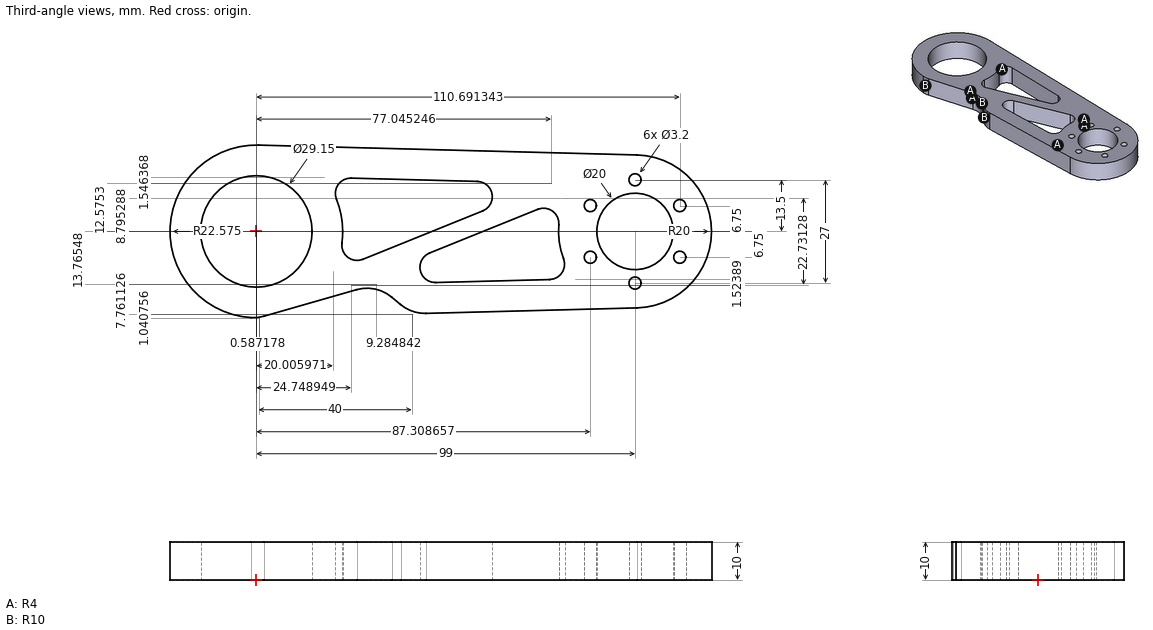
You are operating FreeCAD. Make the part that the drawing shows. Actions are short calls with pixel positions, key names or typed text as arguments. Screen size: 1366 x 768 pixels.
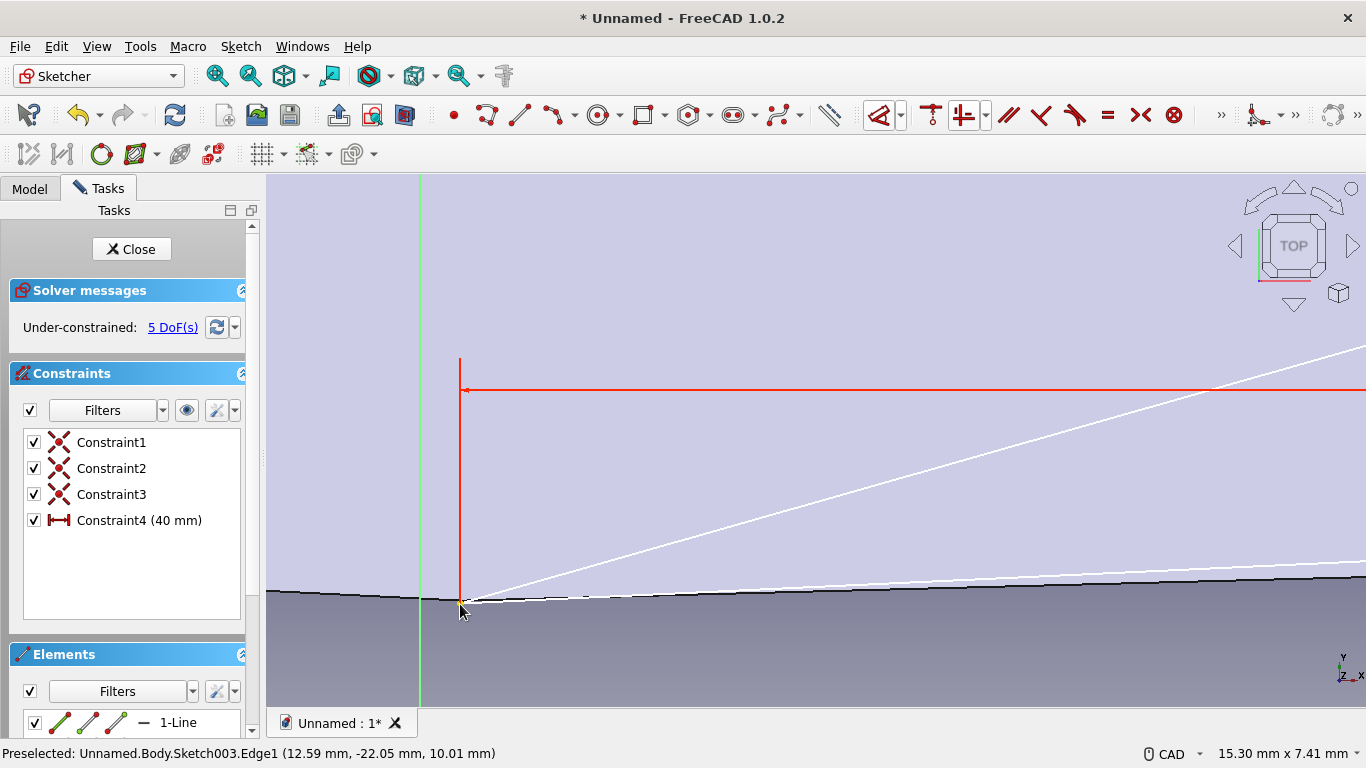
click(460, 604)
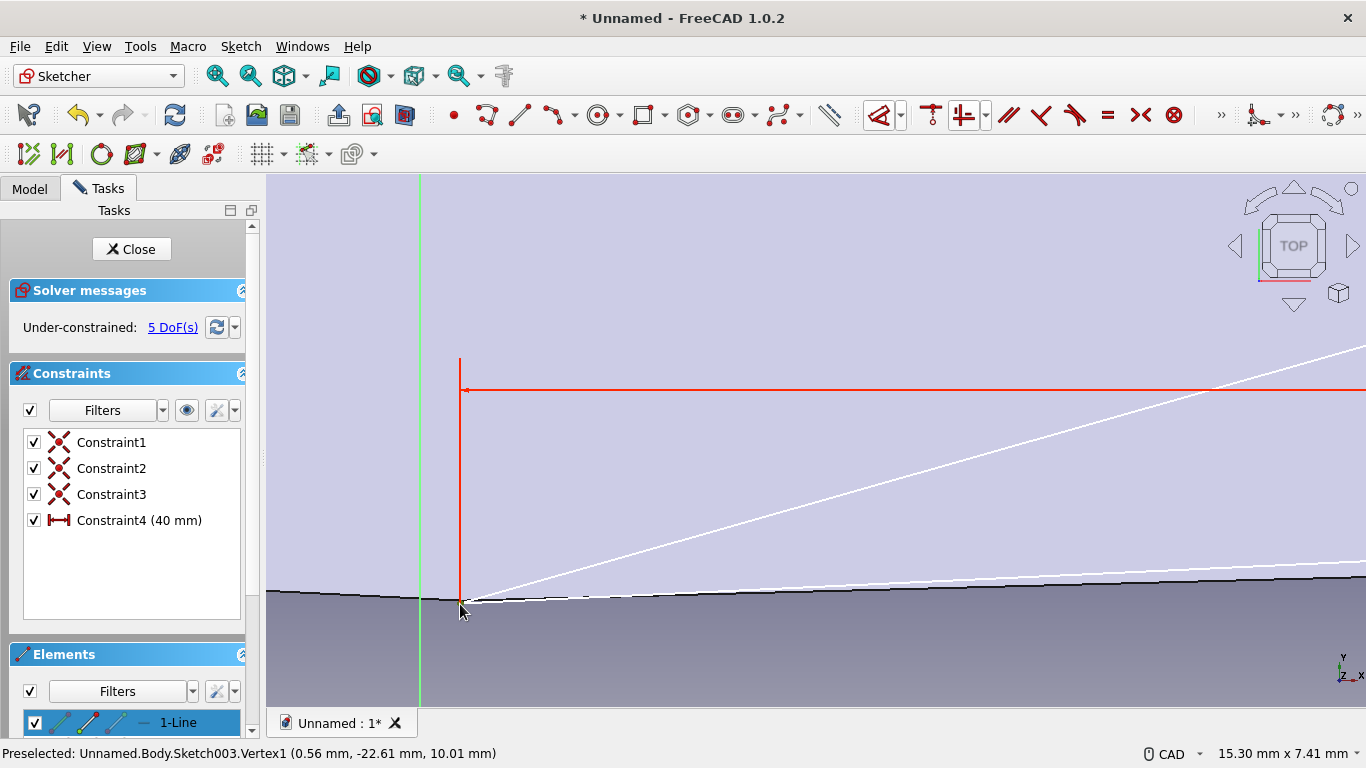
key(l)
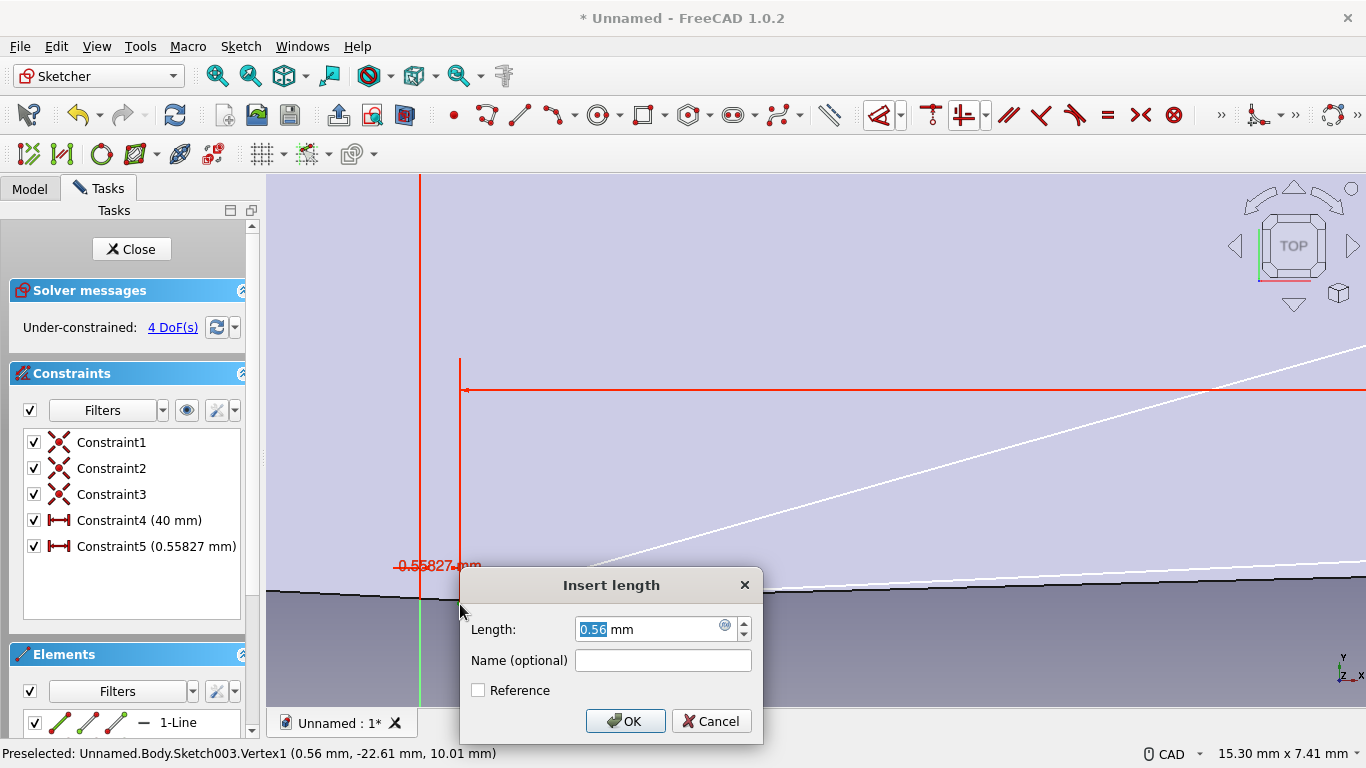
text(0.587178)
key(Return)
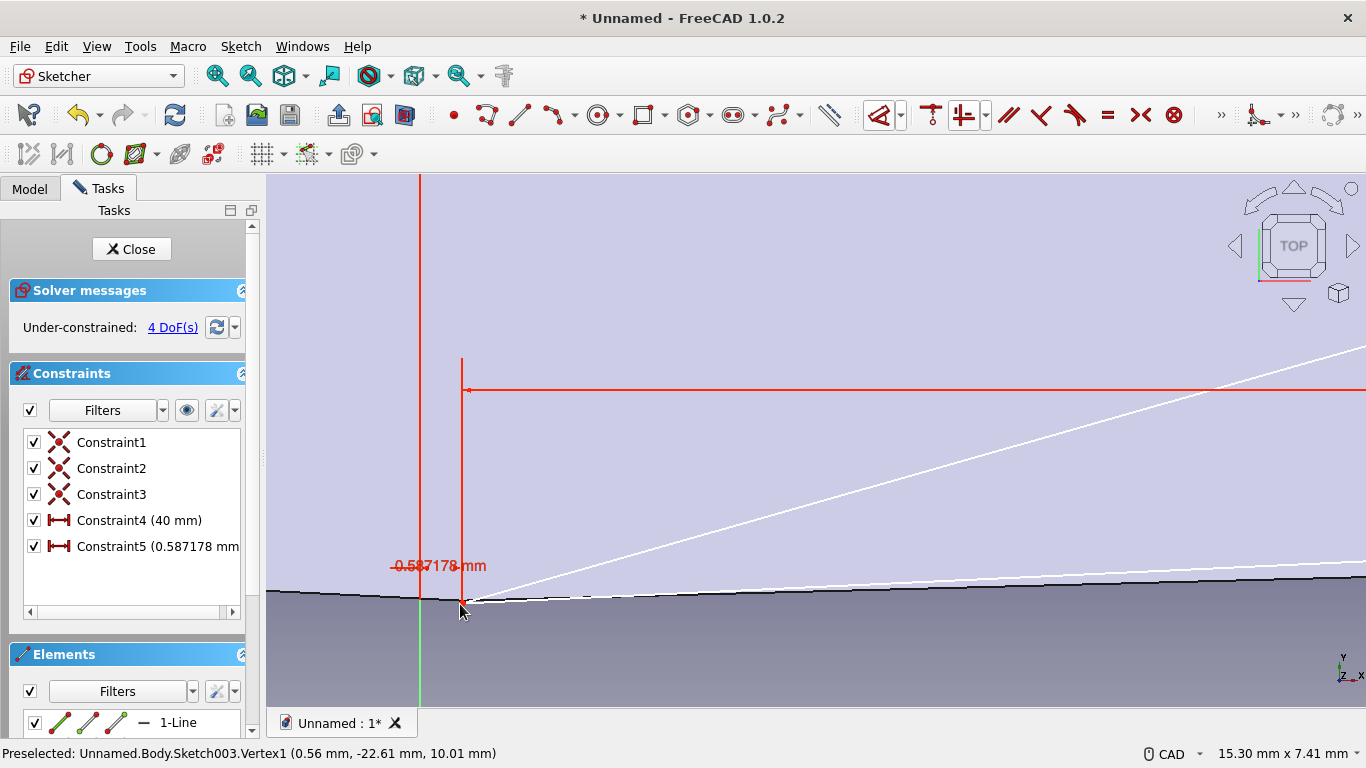
scroll(461, 605, down, 8)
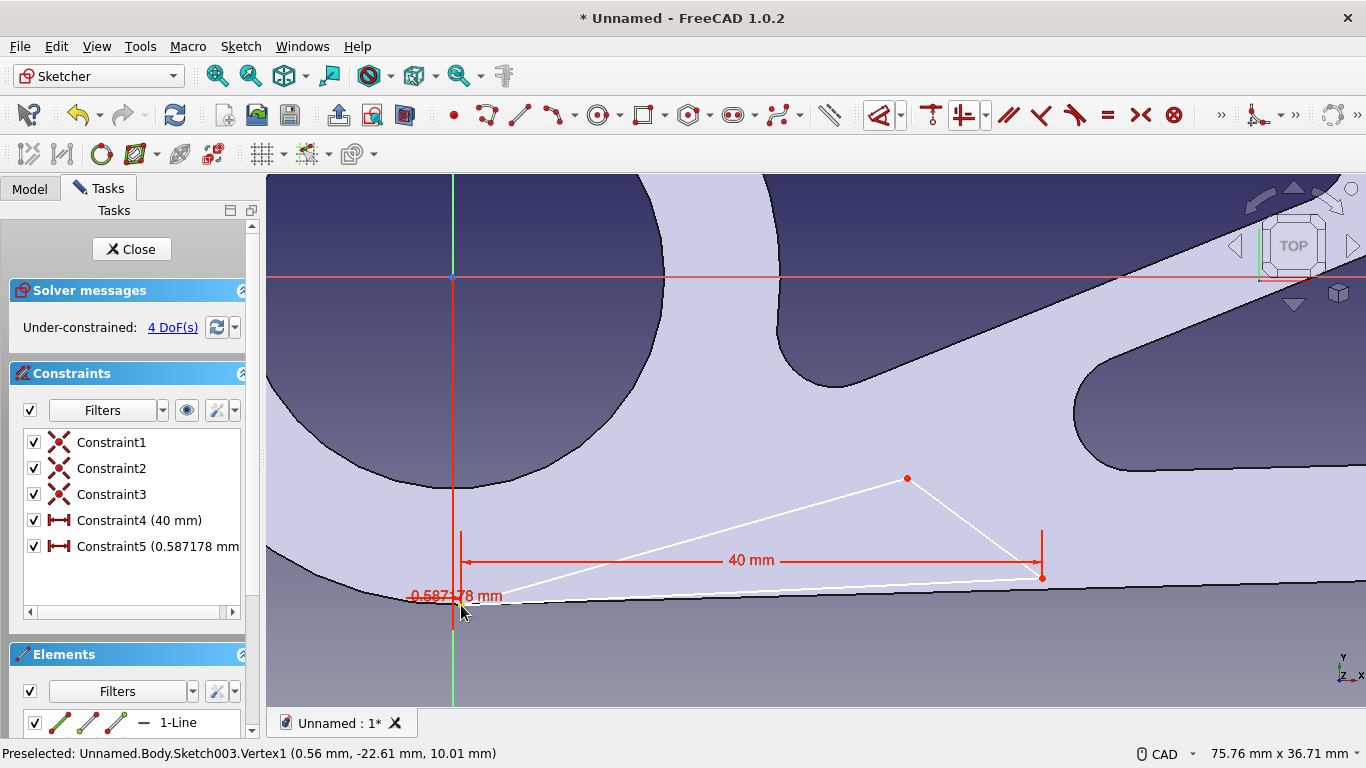
click(908, 478)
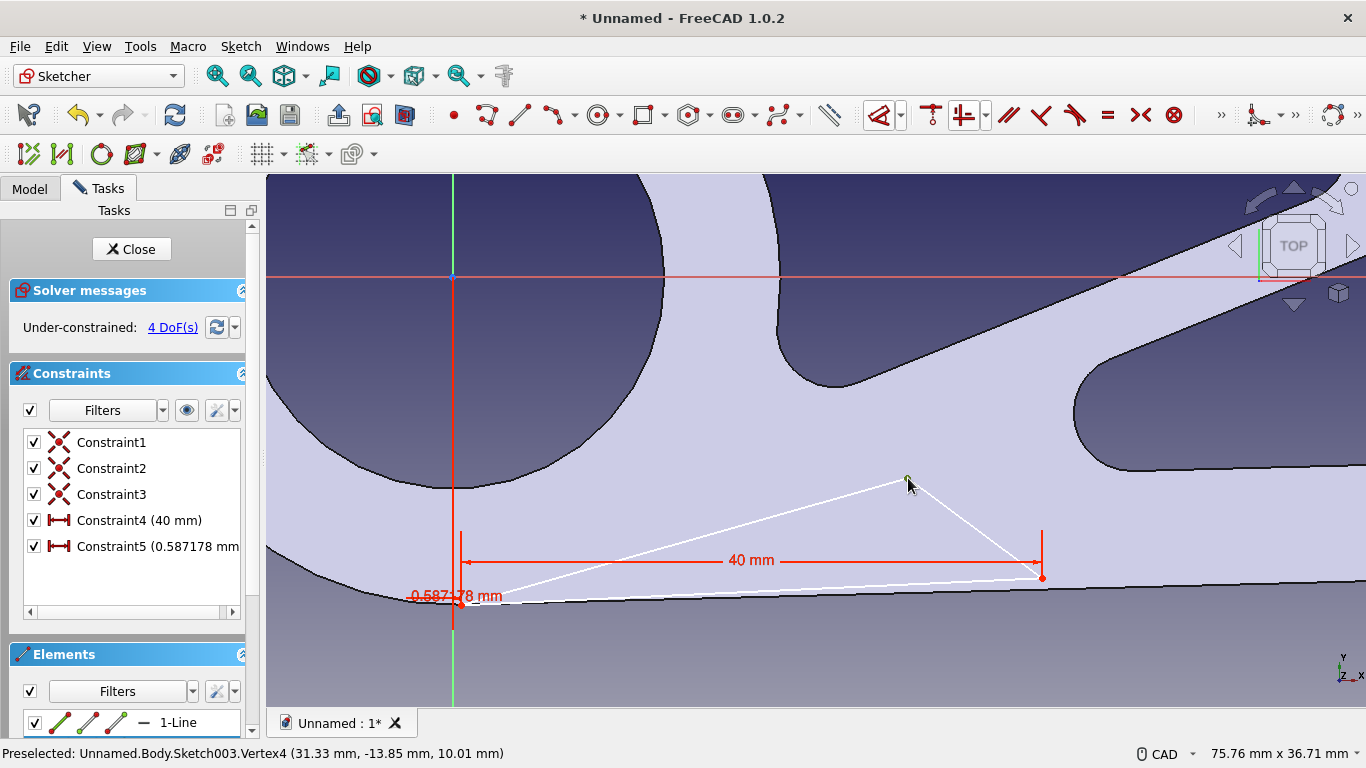
key(i)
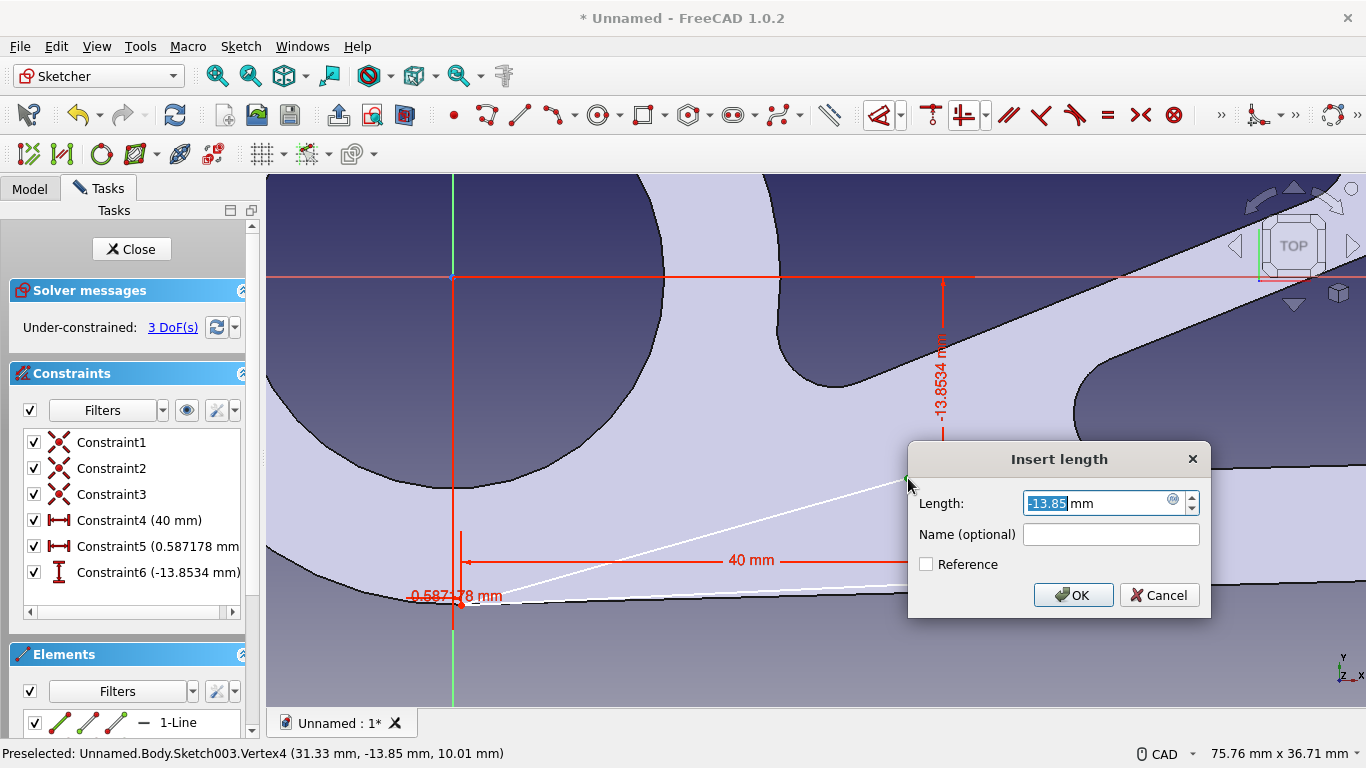
text(-13.76548)
key(Return)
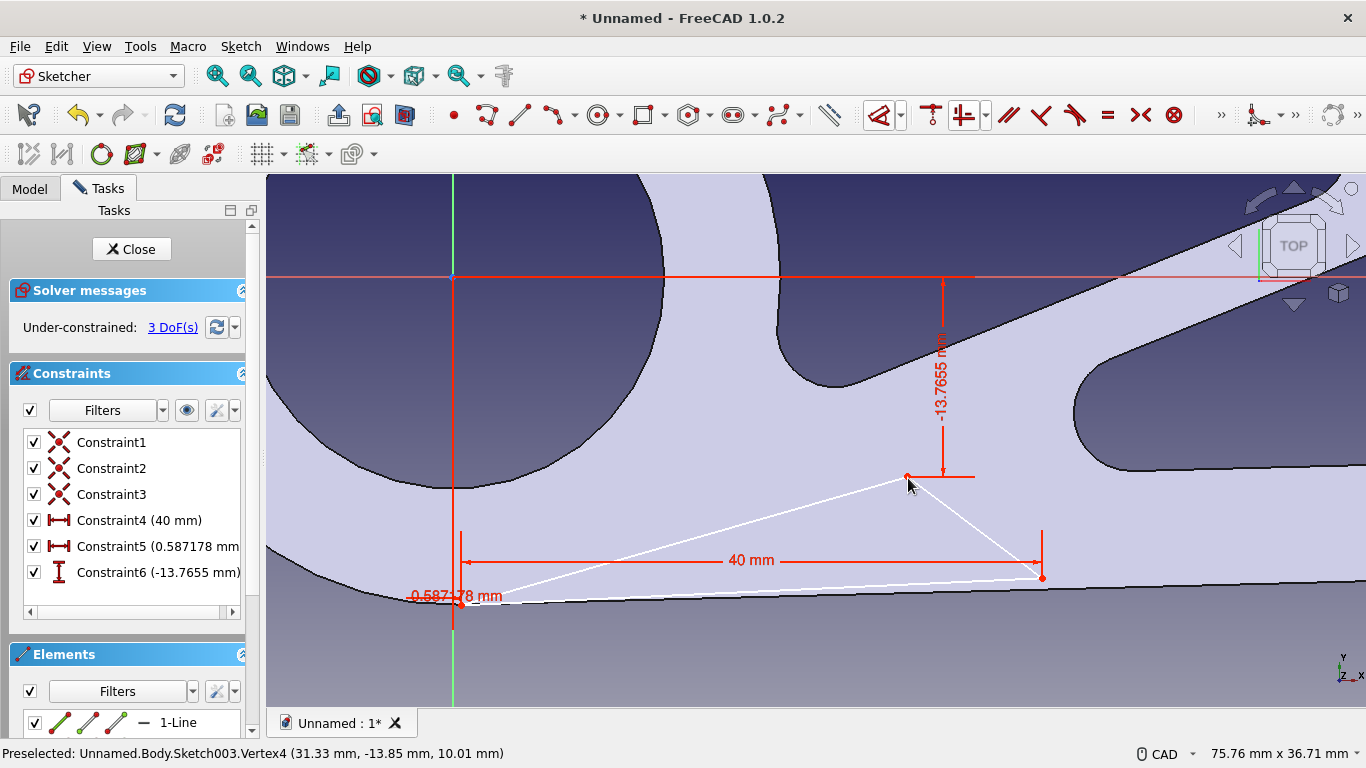
scroll(636, 597, up, 5)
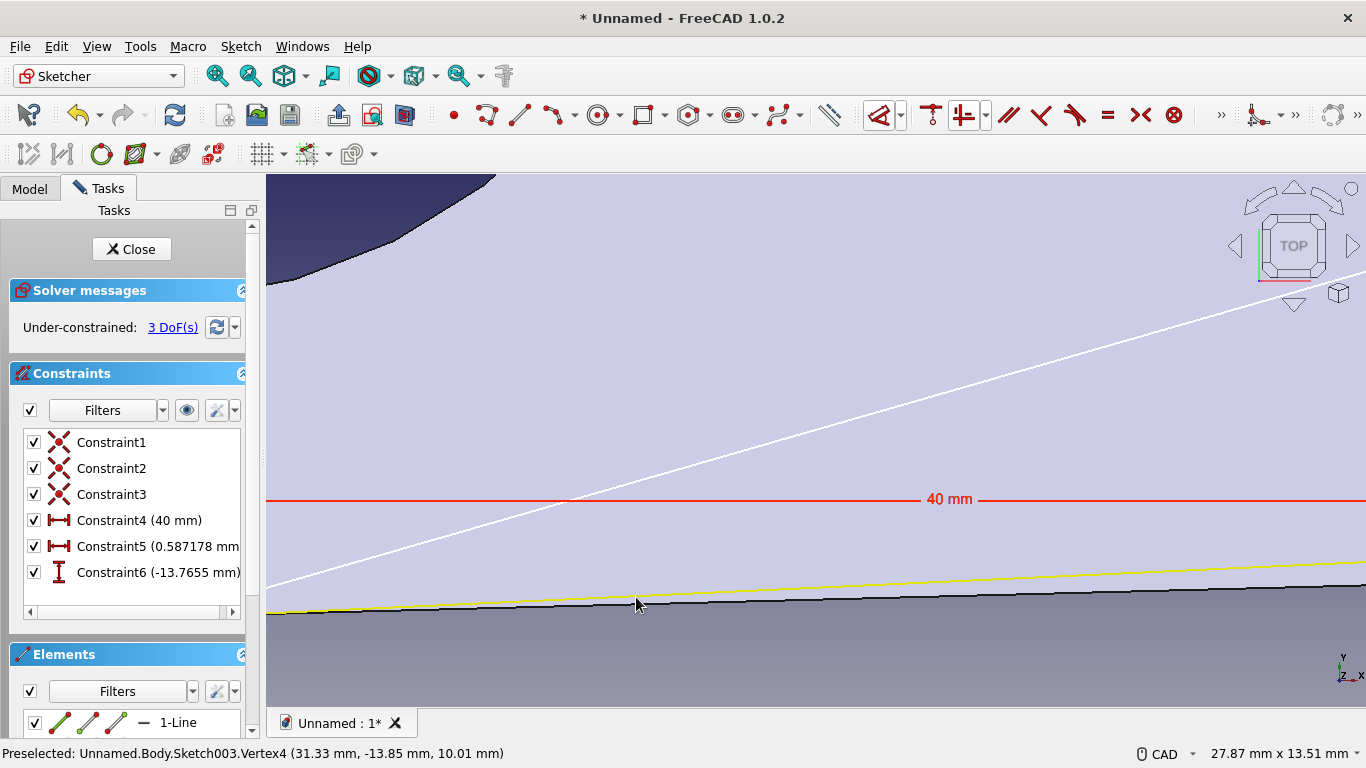
click(634, 596)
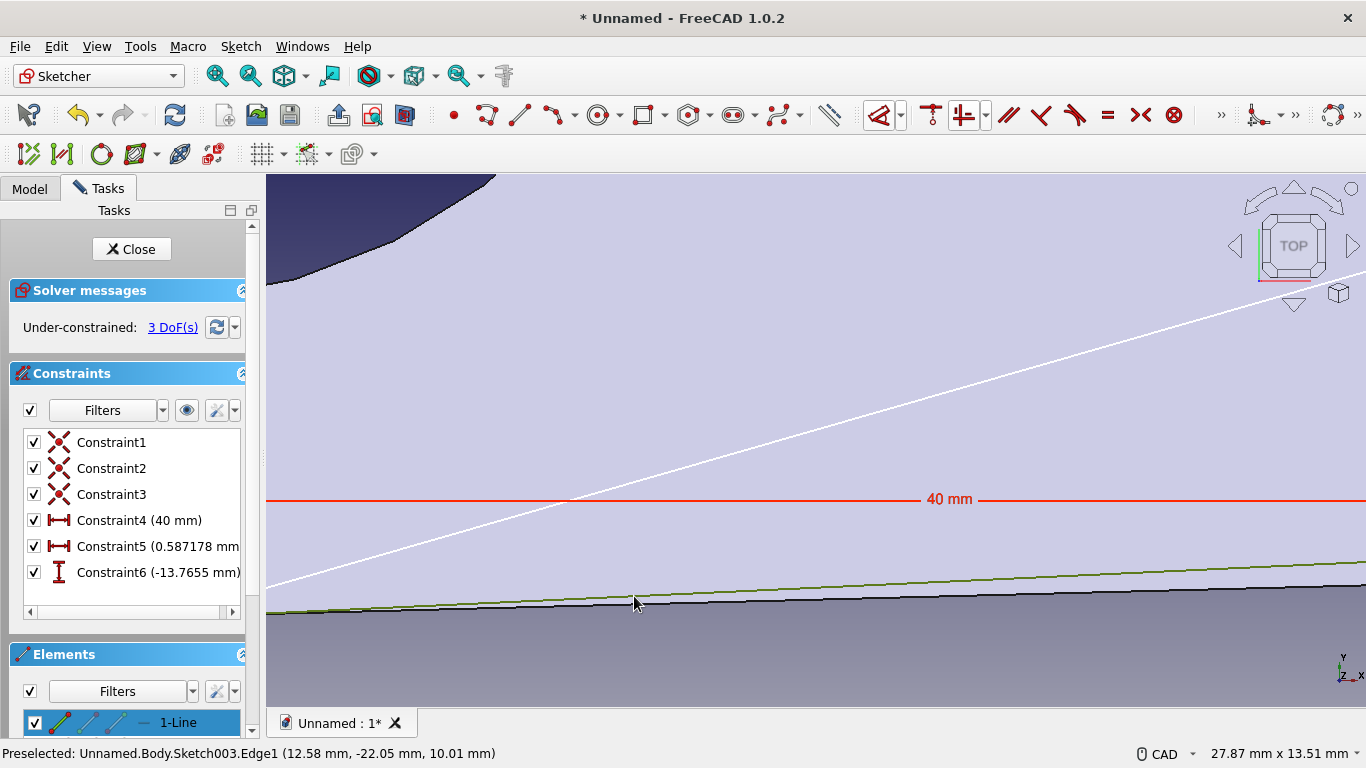
key(i)